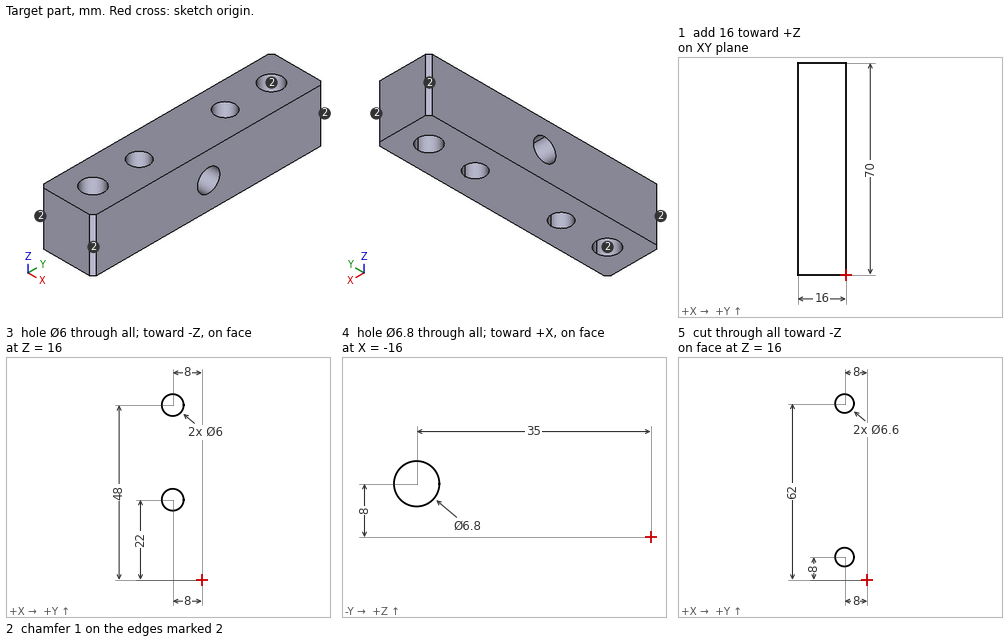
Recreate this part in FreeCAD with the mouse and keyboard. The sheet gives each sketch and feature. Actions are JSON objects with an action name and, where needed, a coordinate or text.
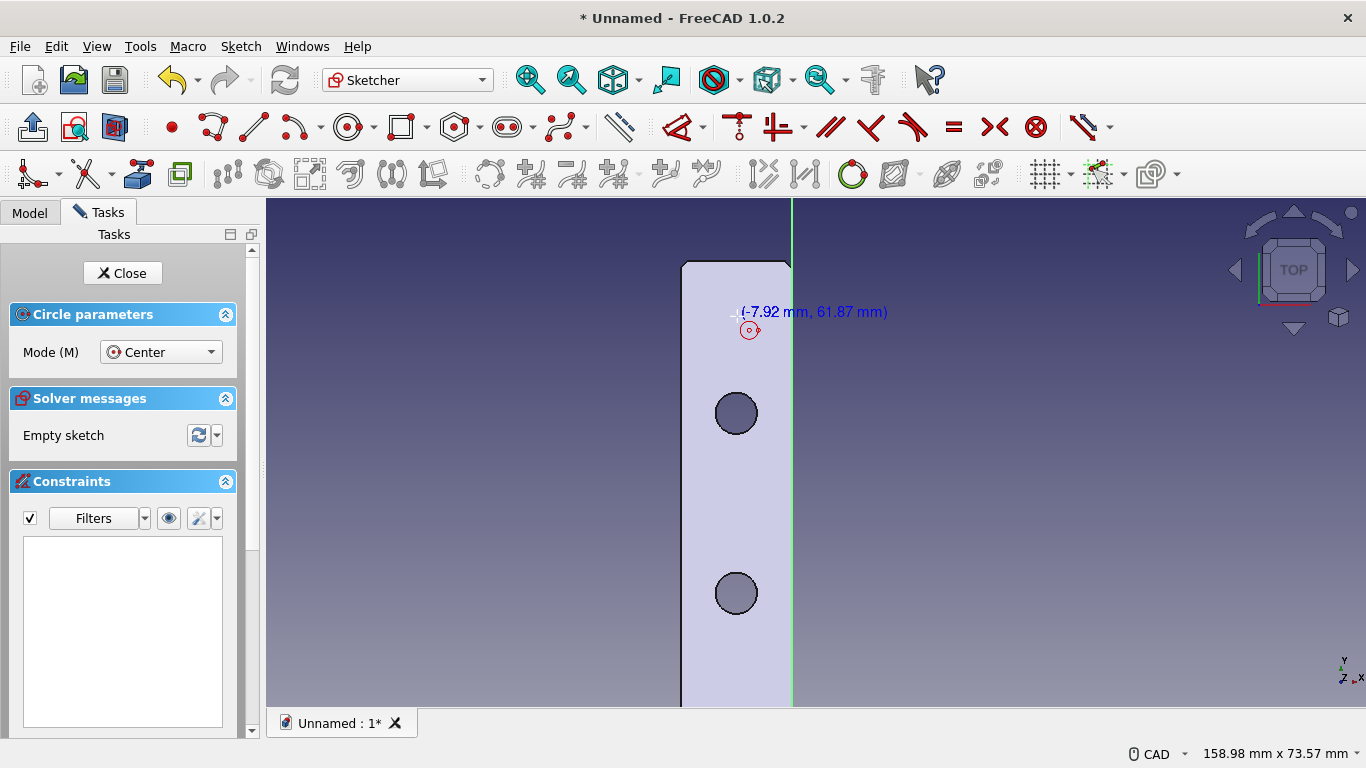
{"action": "left_click", "coordinate": [736, 316]}
{"action": "mouse_move", "coordinate": [752, 300]}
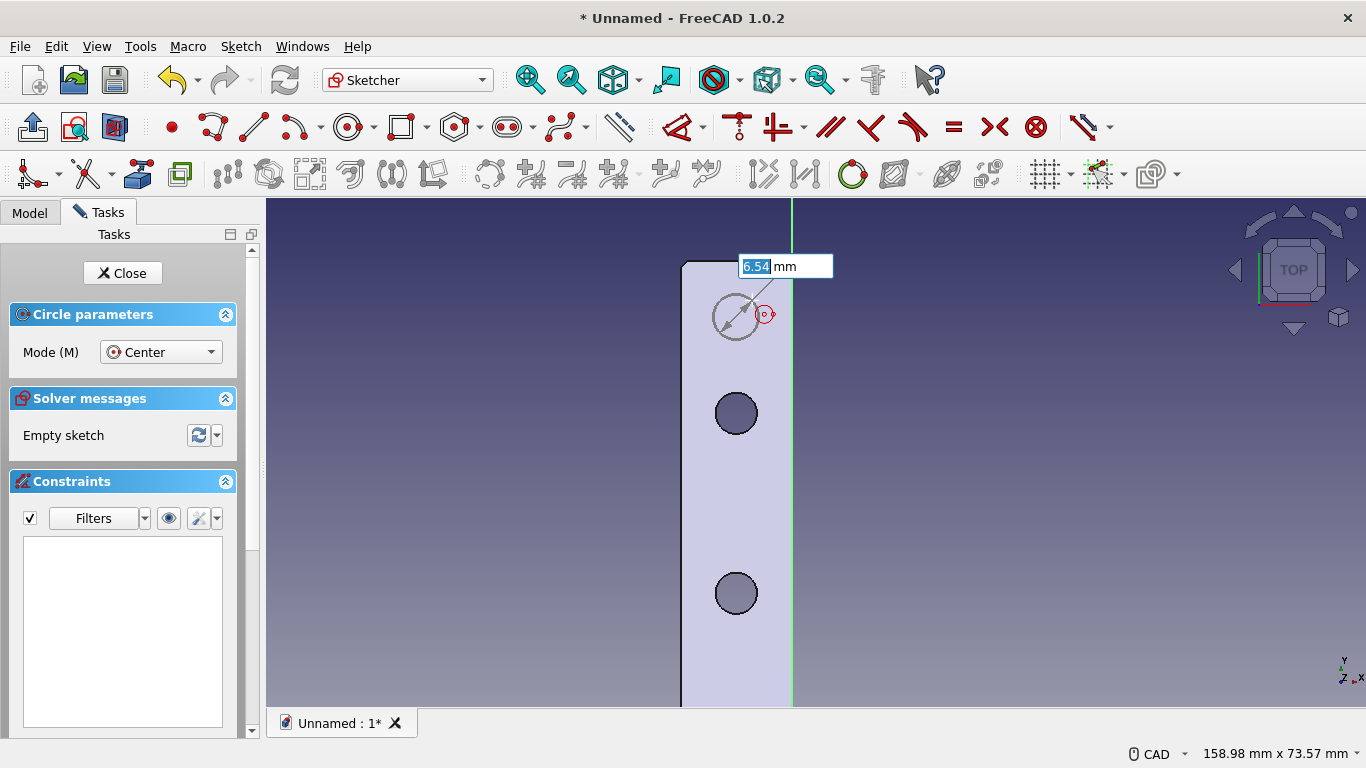
{"action": "type", "text": "6.6"}
{"action": "key", "text": "Return"}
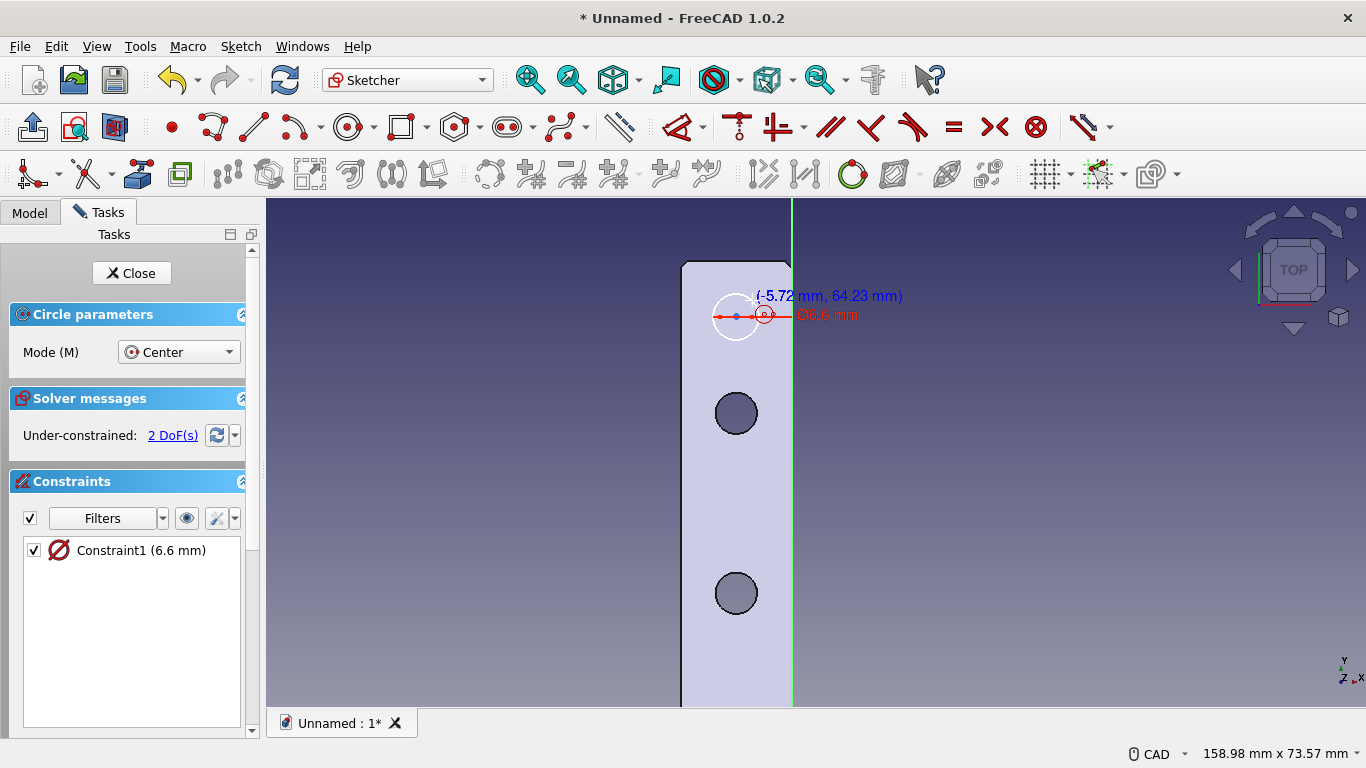
{"action": "scroll", "coordinate": [737, 316], "scroll_direction": "down", "scroll_amount": 2}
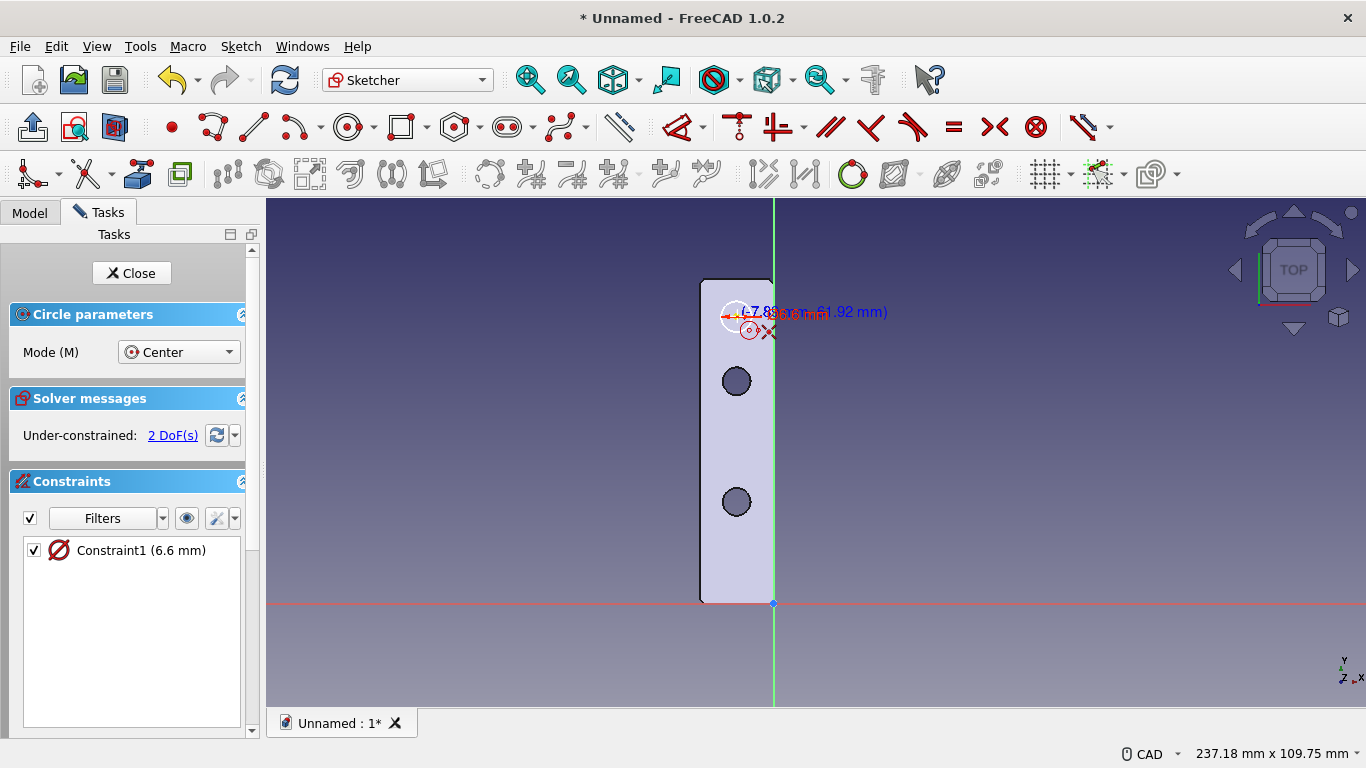
{"action": "scroll", "coordinate": [737, 567], "scroll_direction": "up", "scroll_amount": 2}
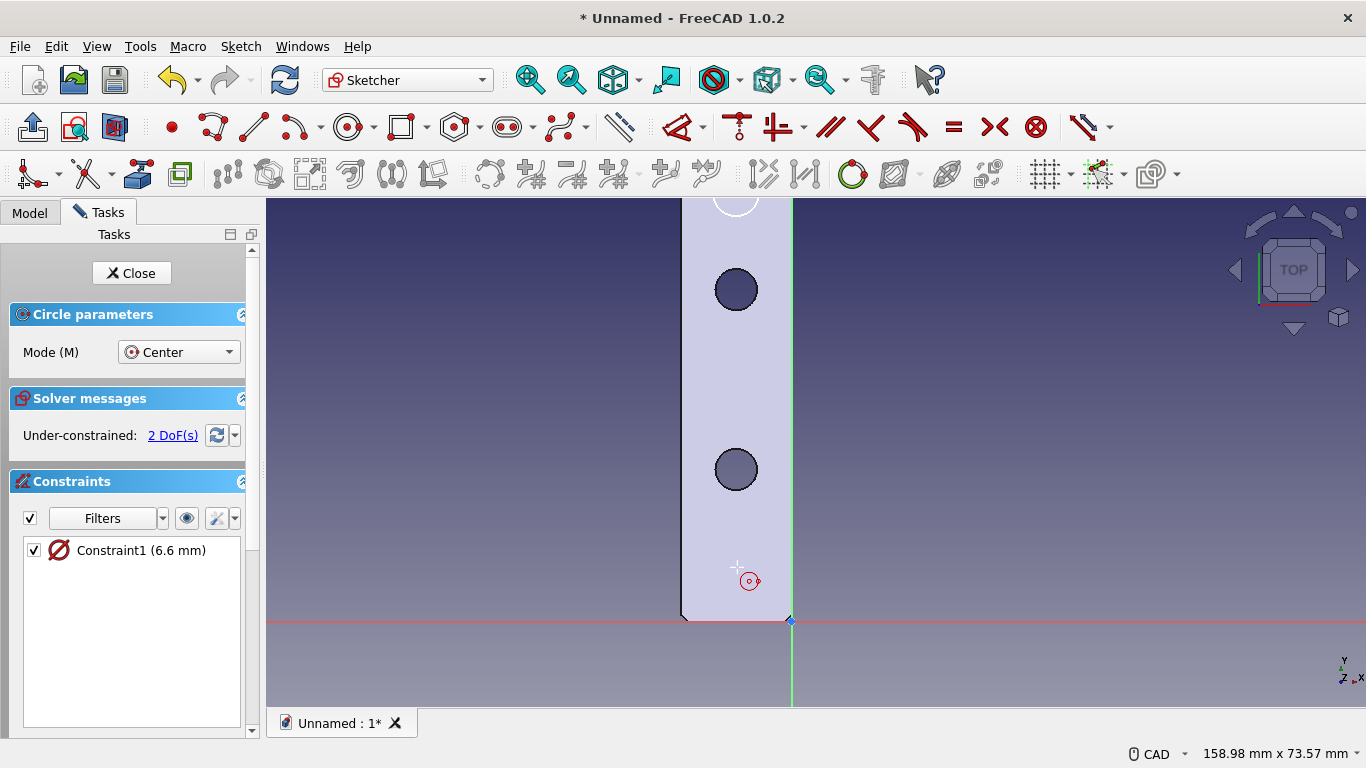
{"action": "left_click", "coordinate": [736, 566]}
{"action": "mouse_move", "coordinate": [752, 550]}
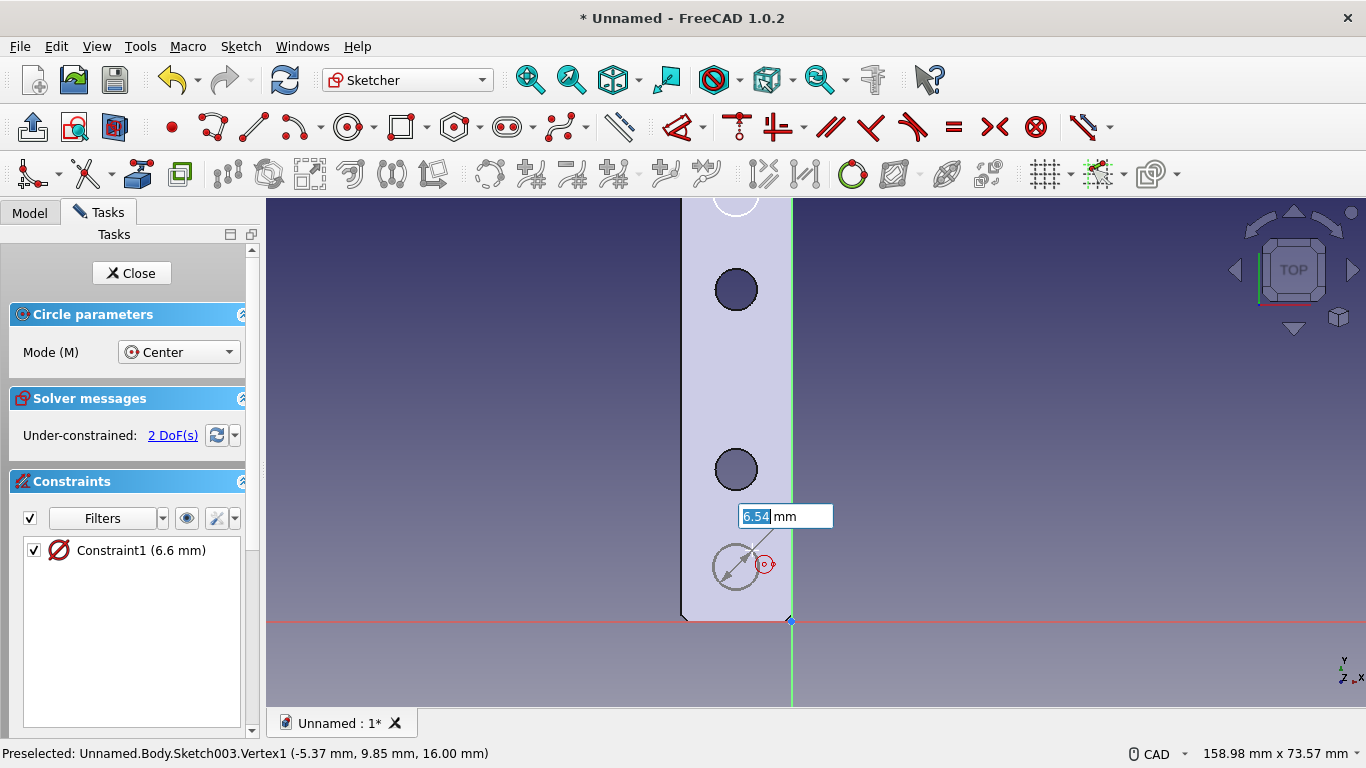
{"action": "type", "text": "6.6"}
{"action": "key", "text": "Return"}
{"action": "key", "text": "Escape"}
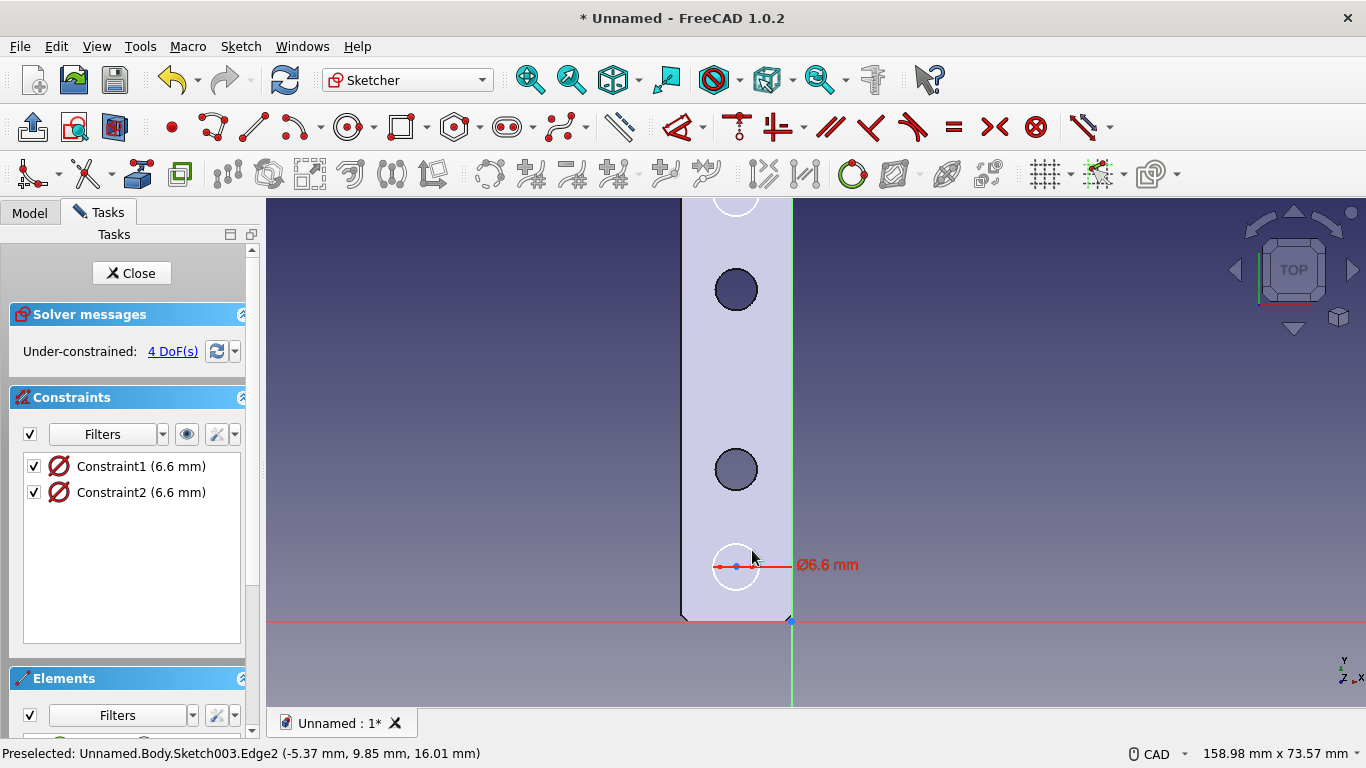
{"action": "left_click", "coordinate": [676, 128]}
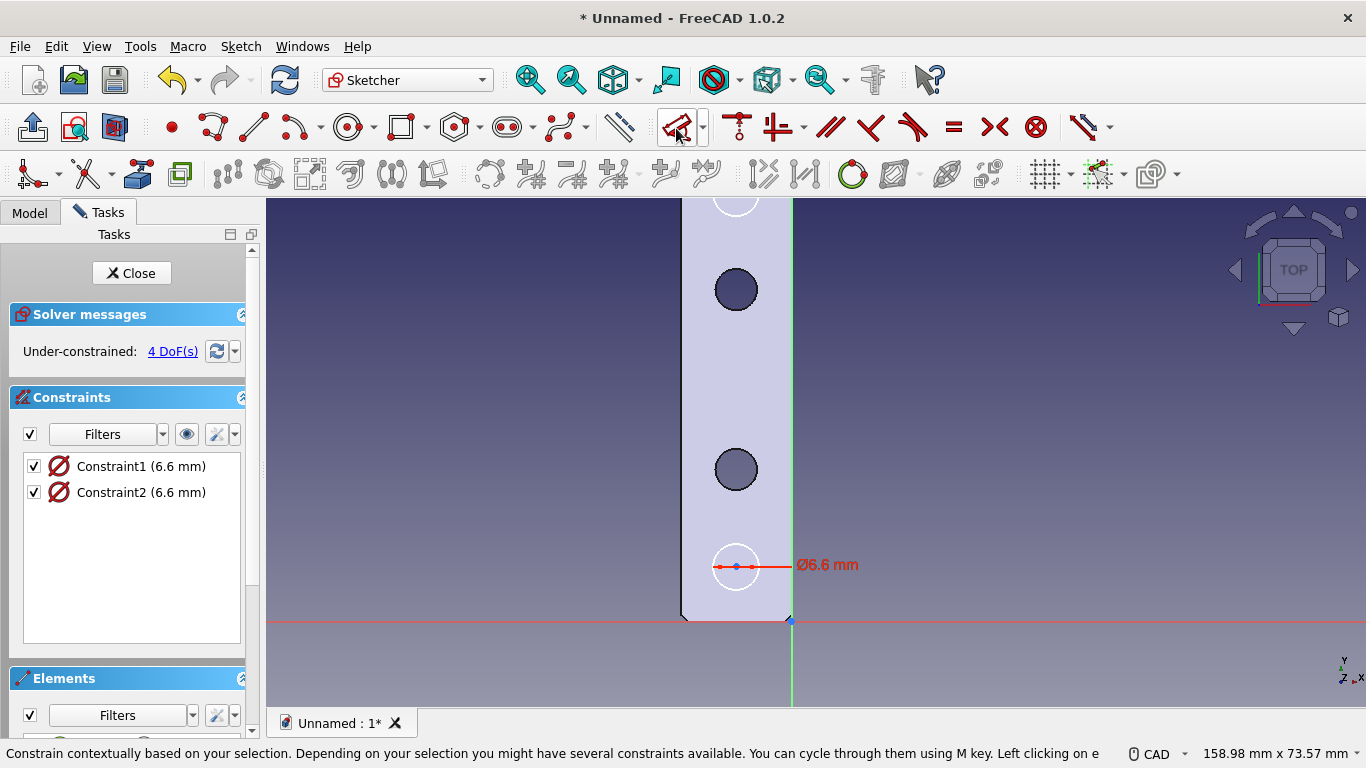
{"action": "scroll", "coordinate": [737, 568], "scroll_direction": "down", "scroll_amount": 2}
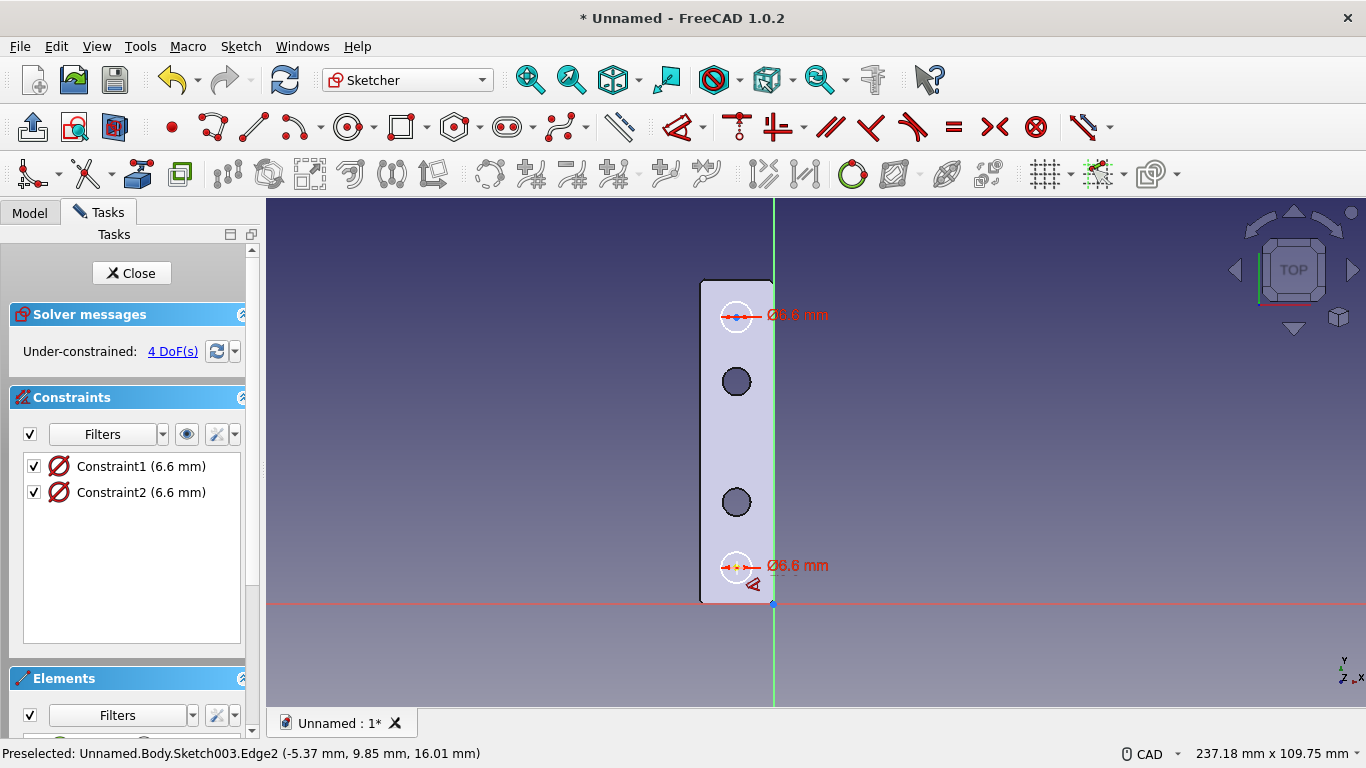
{"action": "left_click", "coordinate": [736, 317]}
{"action": "left_click", "coordinate": [755, 638]}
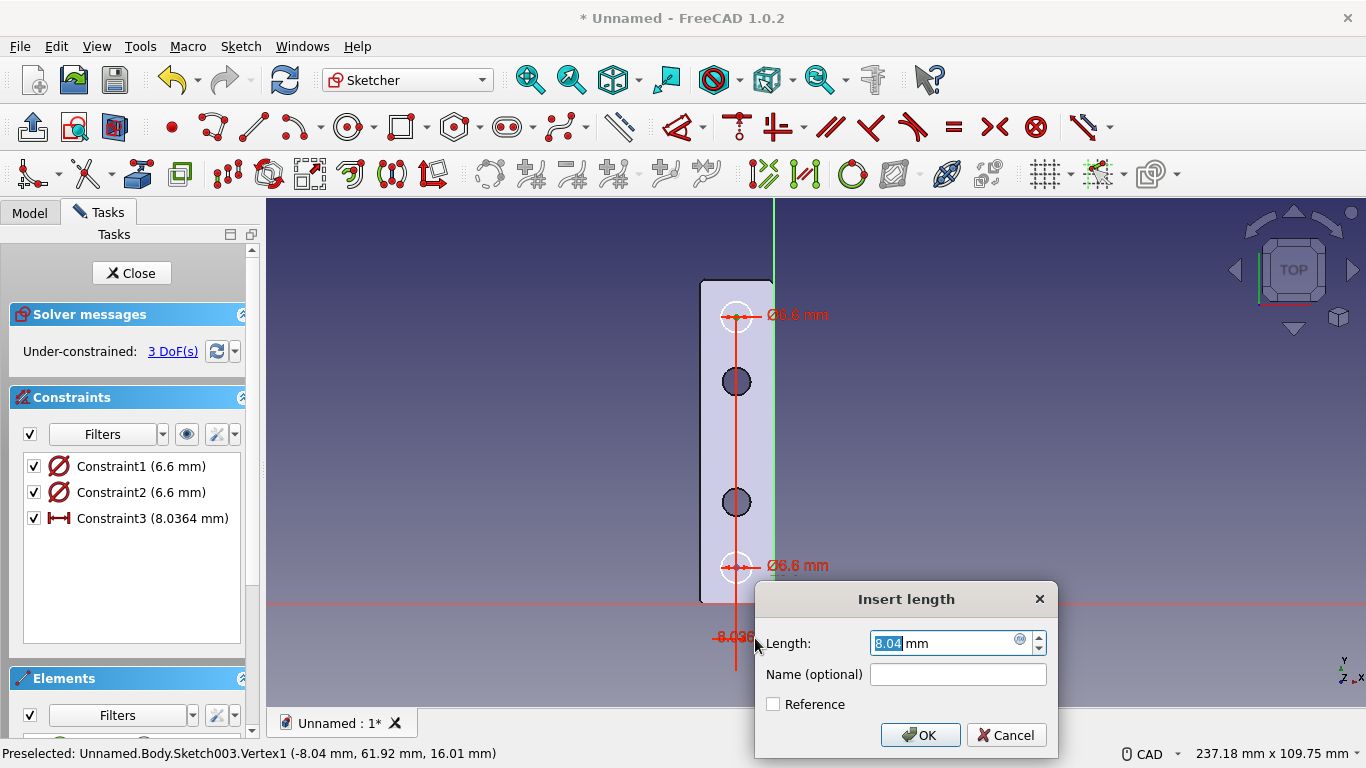
{"action": "type", "text": "8"}
{"action": "key", "text": "Return"}